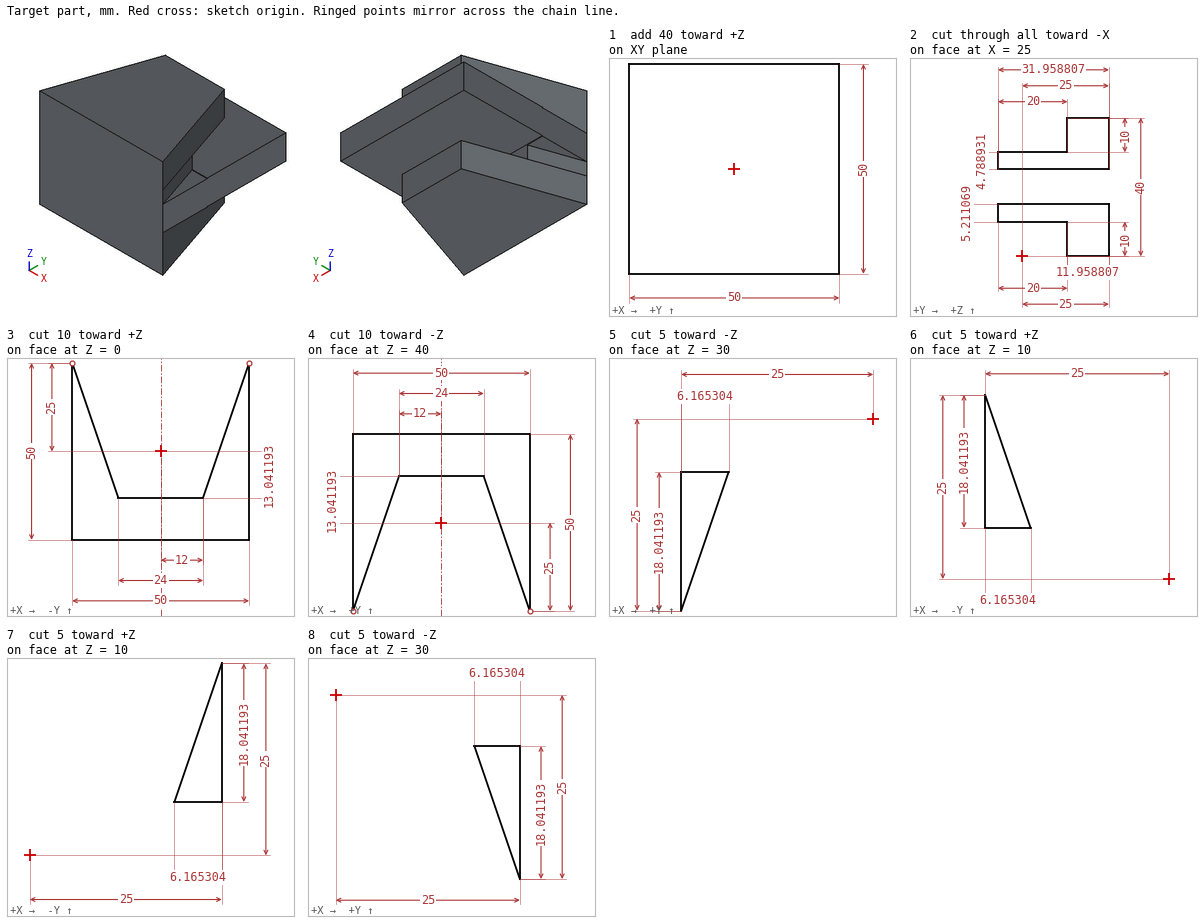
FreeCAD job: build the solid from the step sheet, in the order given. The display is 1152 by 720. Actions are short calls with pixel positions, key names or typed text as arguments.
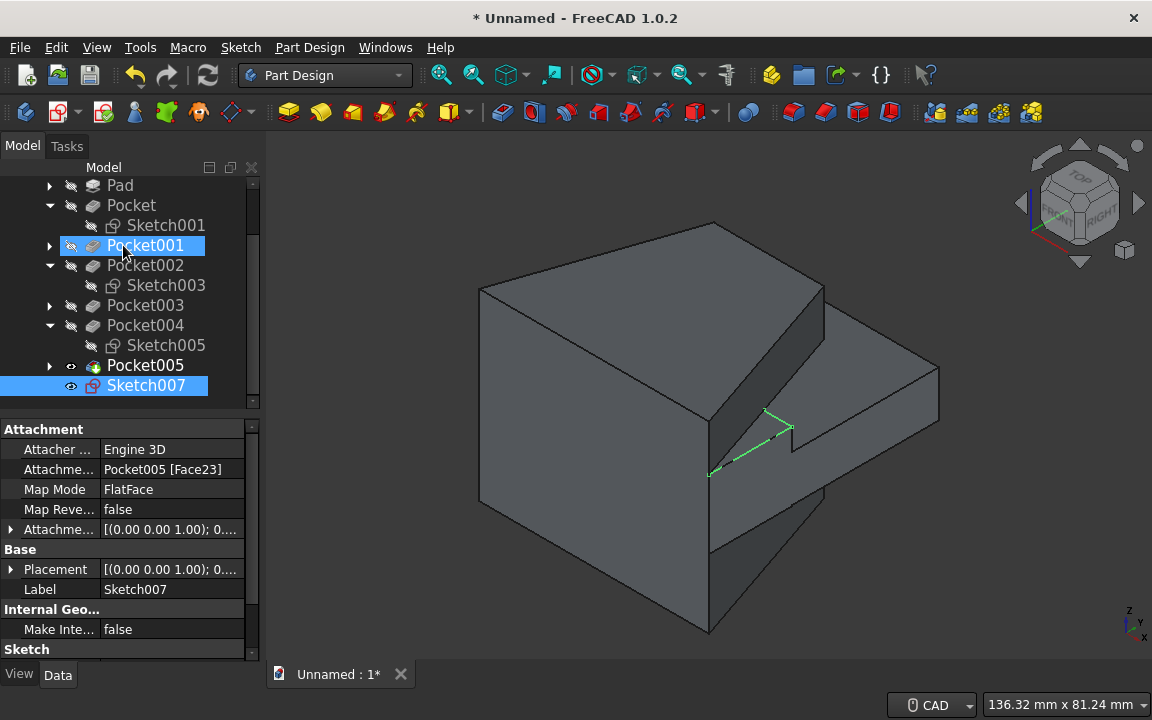
click(504, 112)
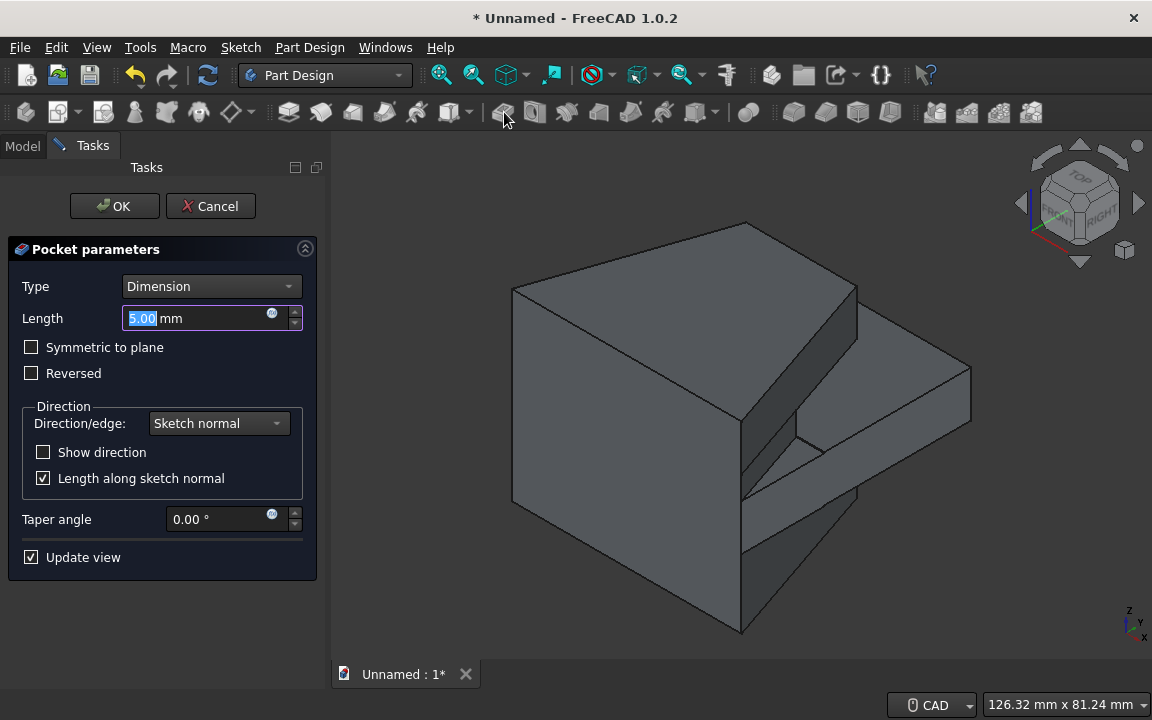
text(5)
key(Tab)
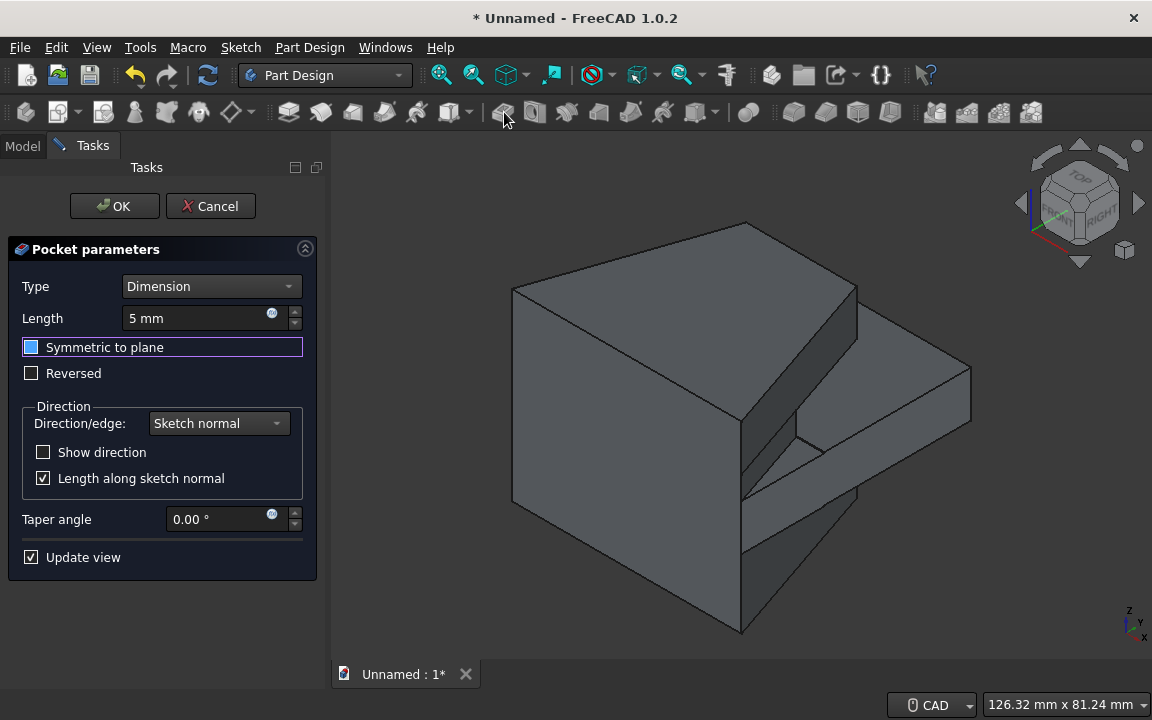
click(115, 206)